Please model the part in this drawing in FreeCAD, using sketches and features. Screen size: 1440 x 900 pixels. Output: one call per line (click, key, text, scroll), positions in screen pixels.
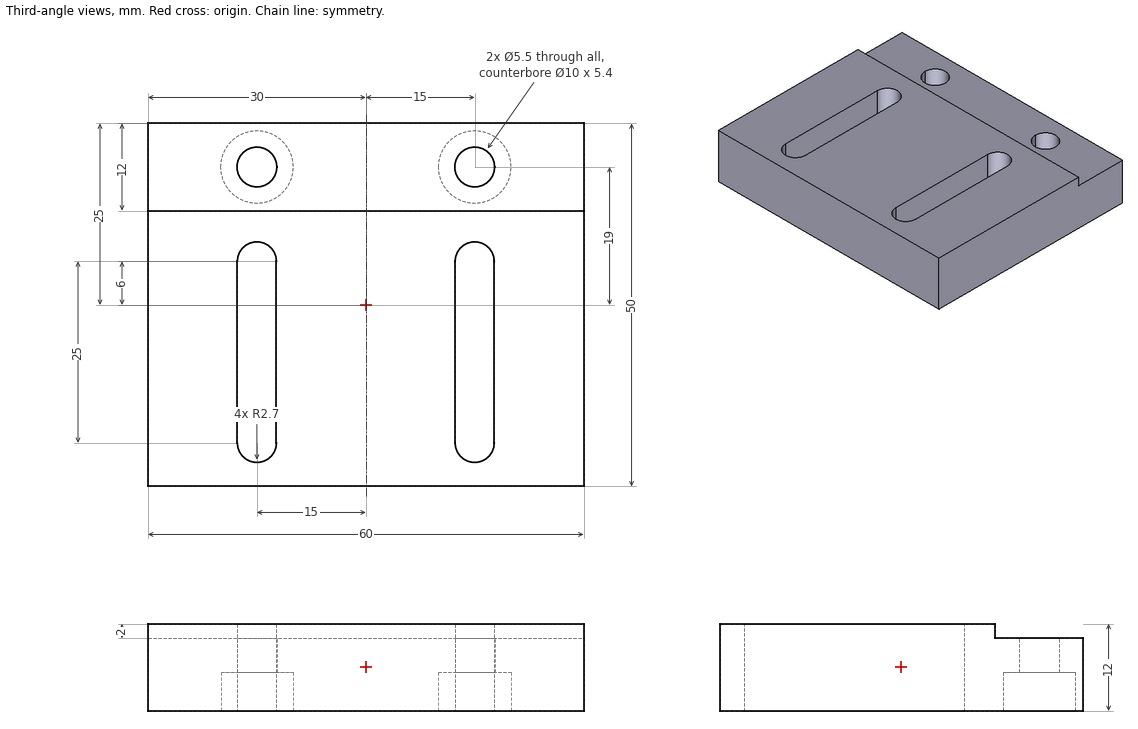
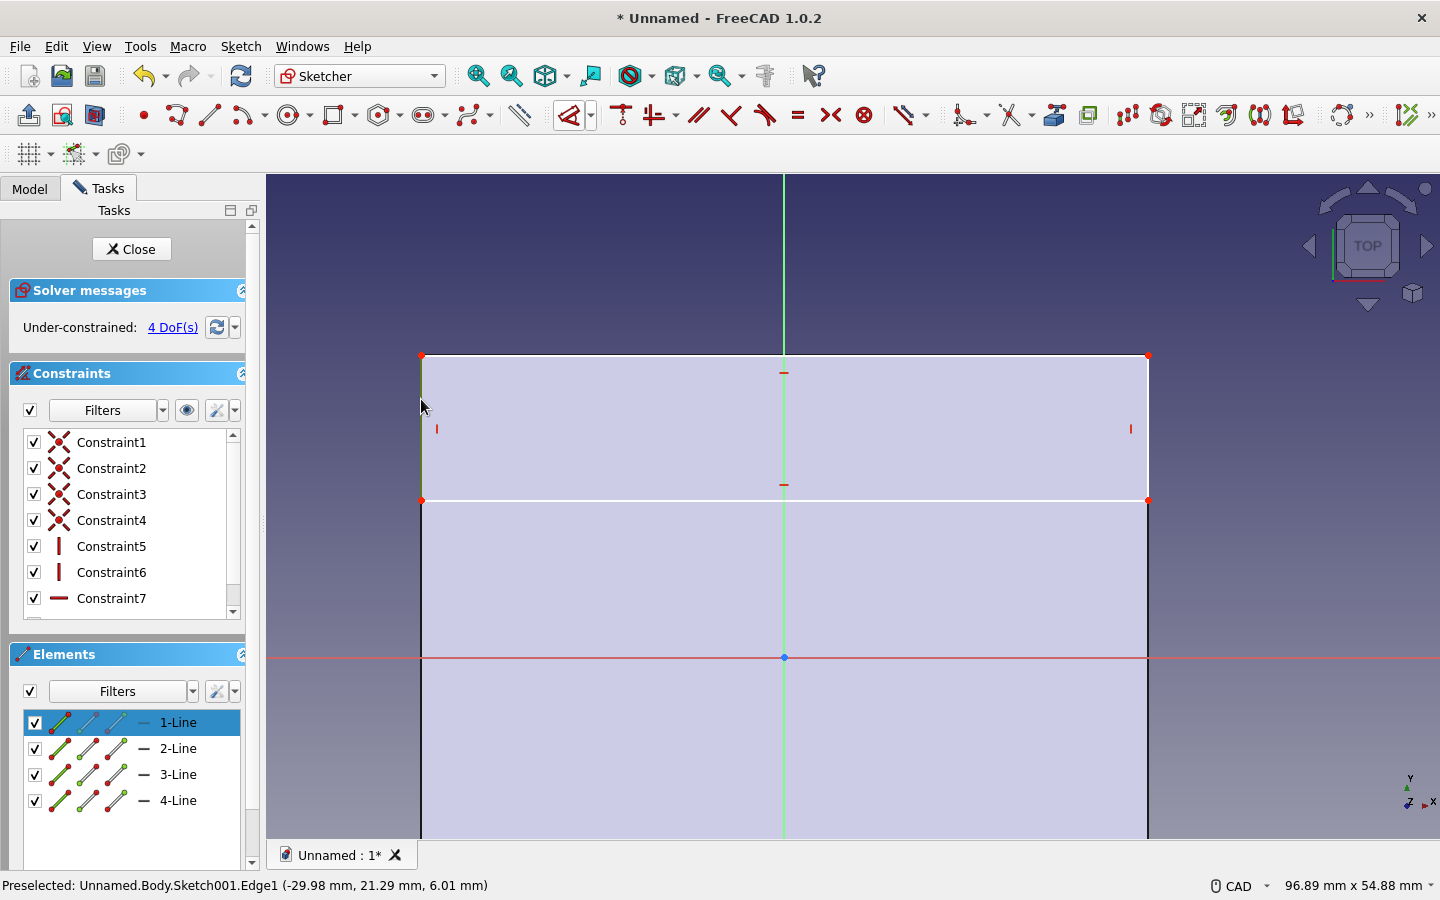
click(590, 116)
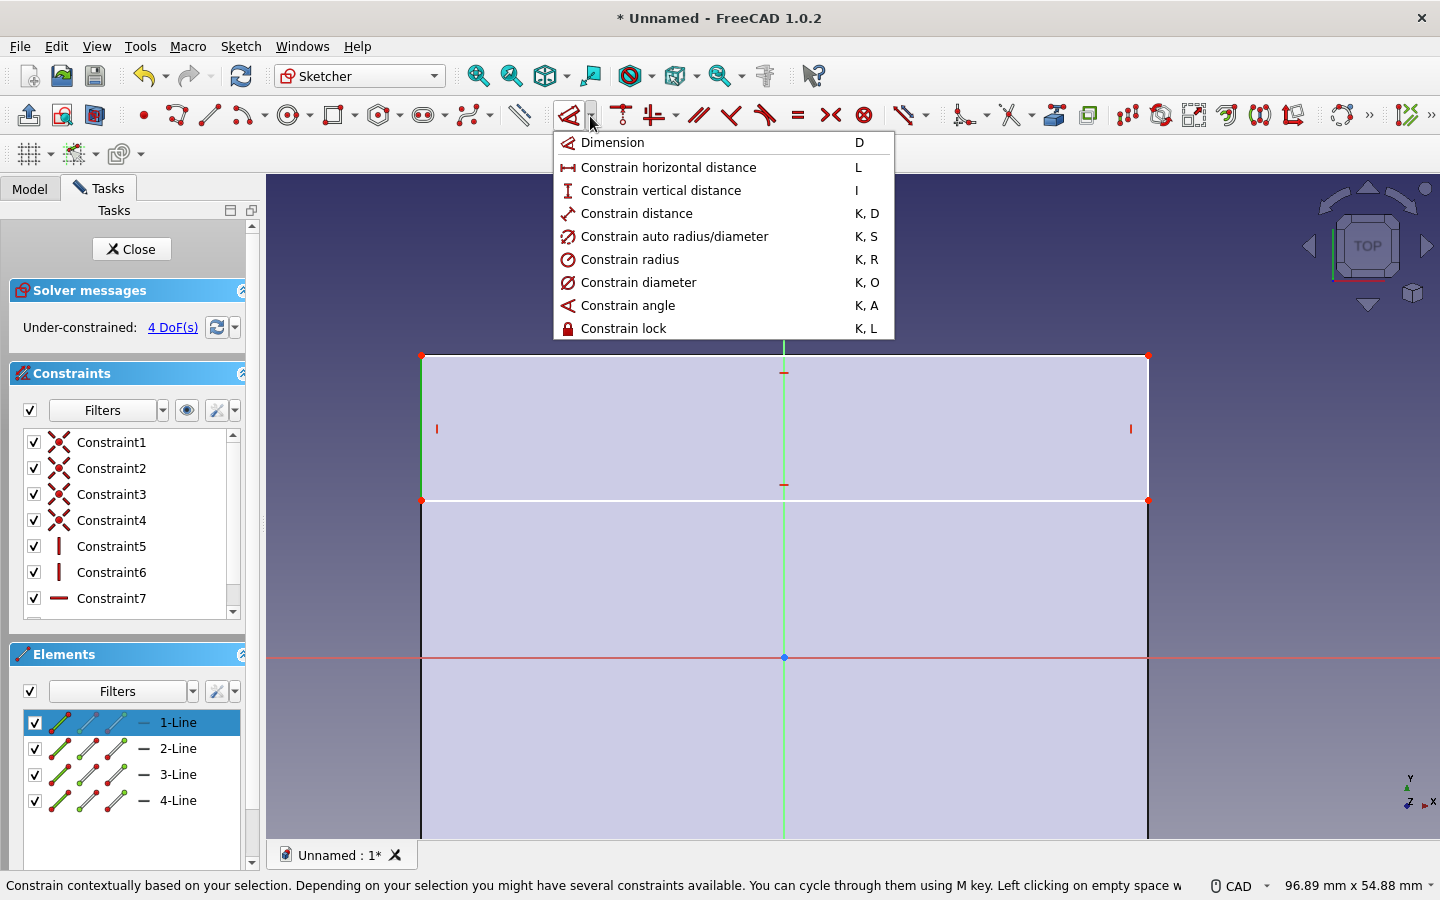
click(724, 190)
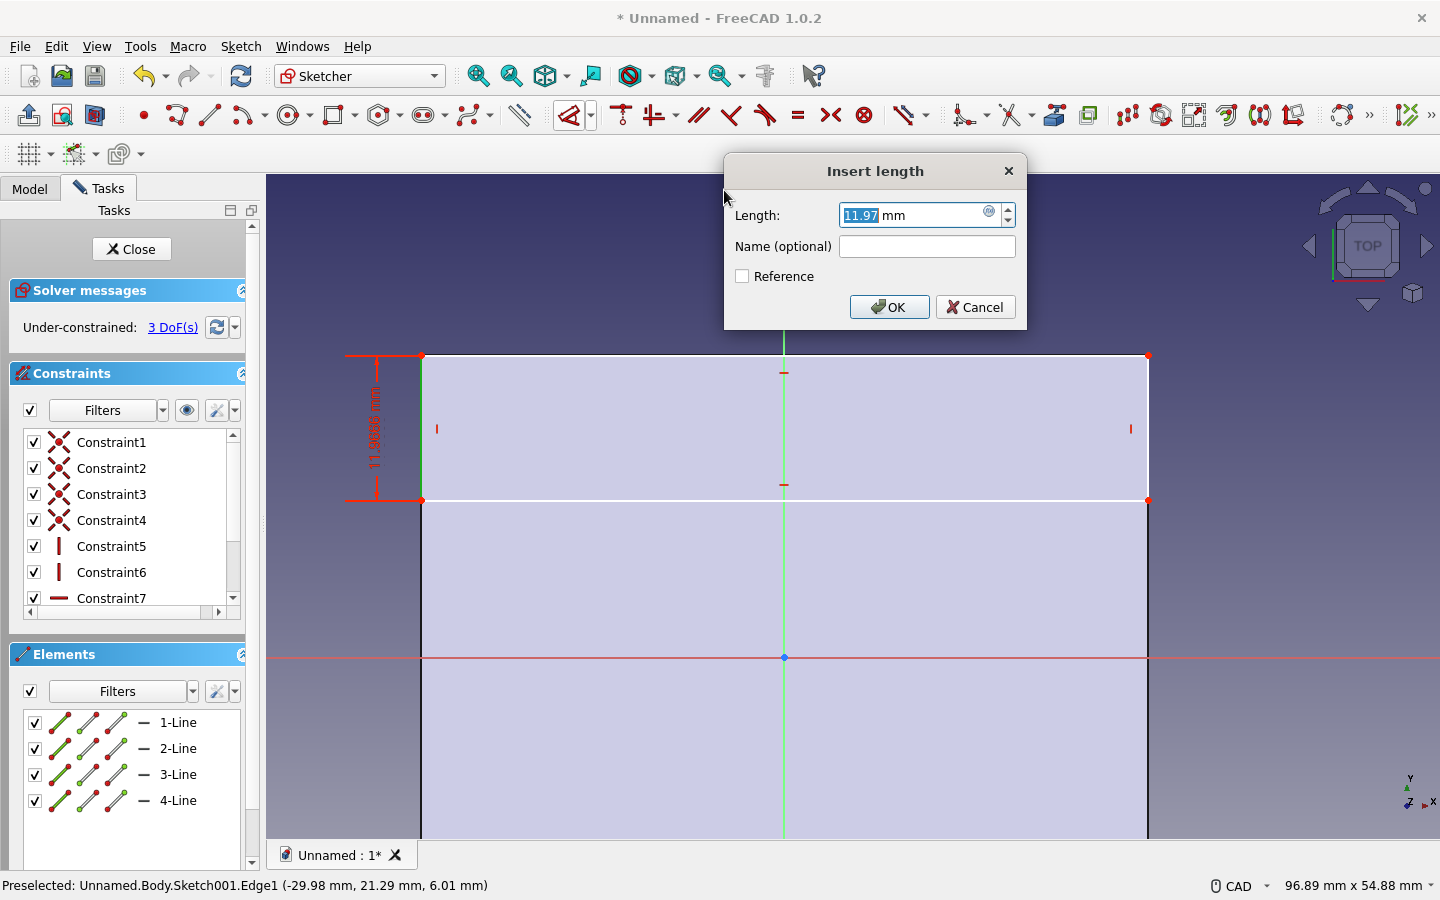
text(12)
key(Return)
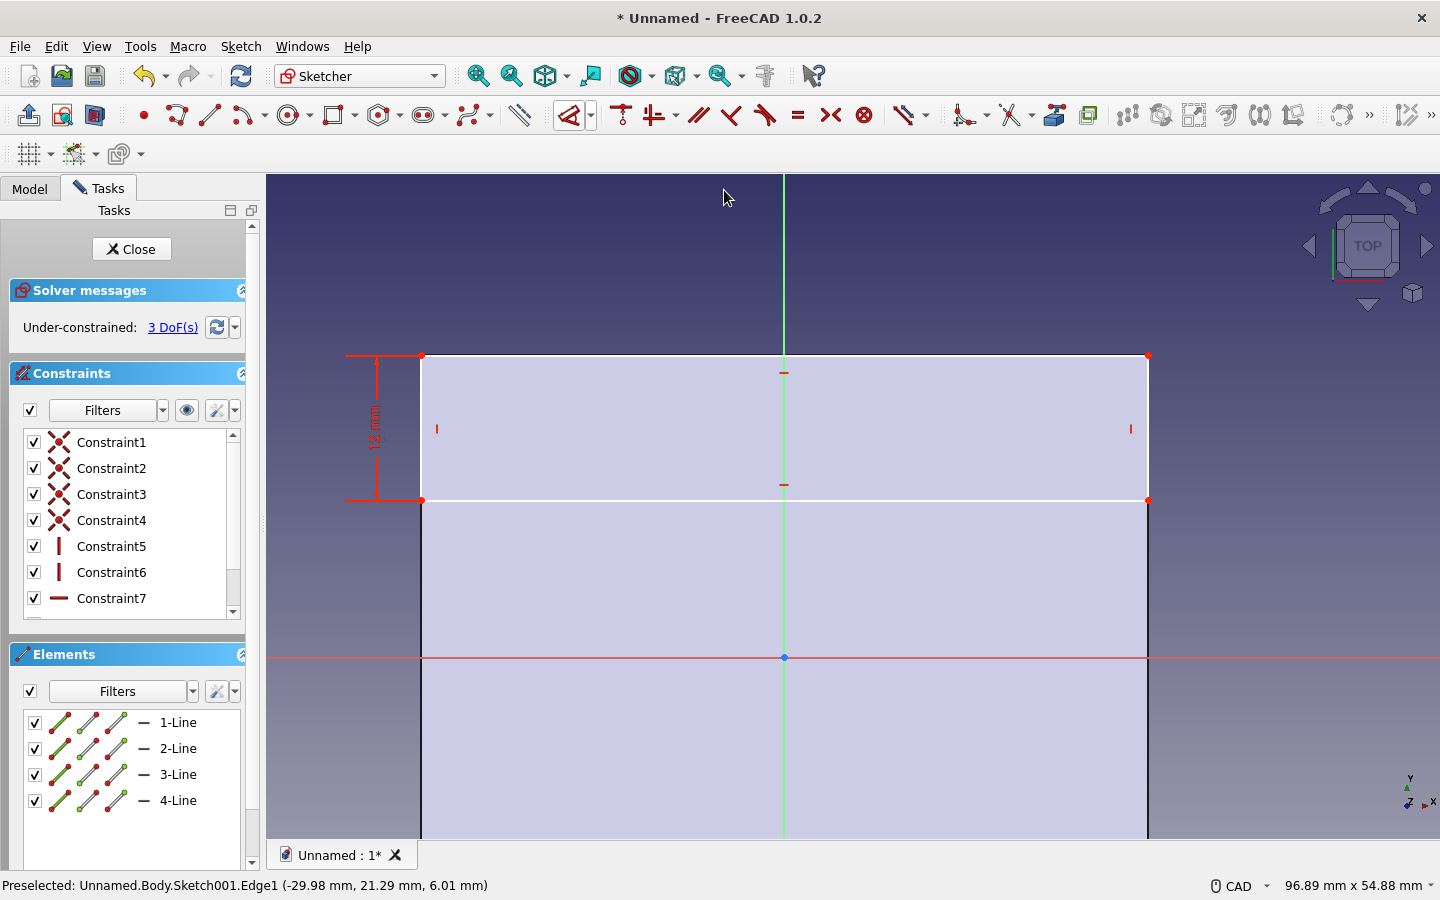
click(639, 501)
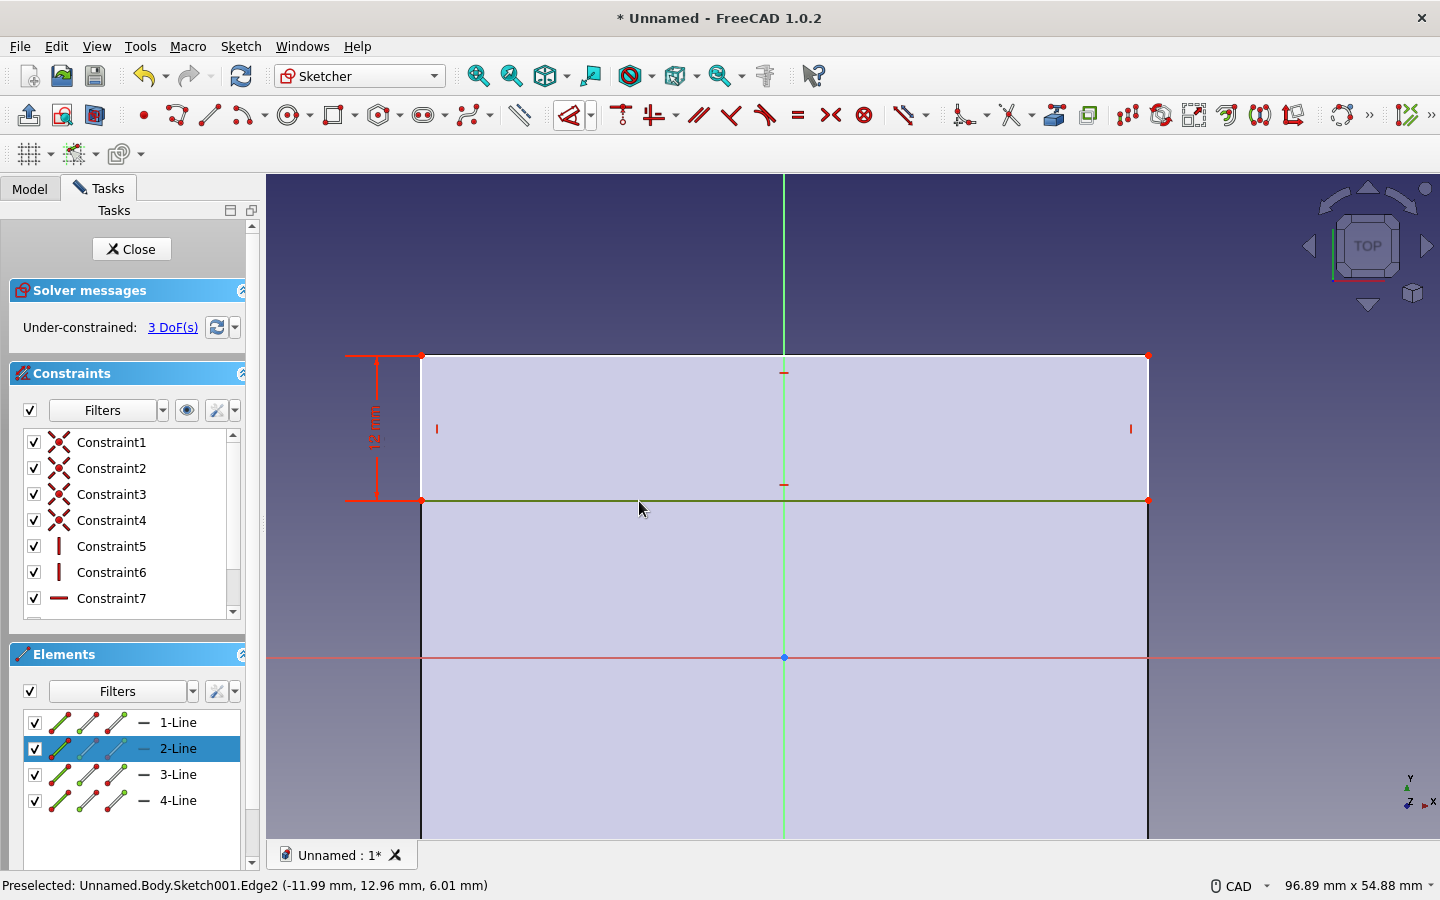
key(l)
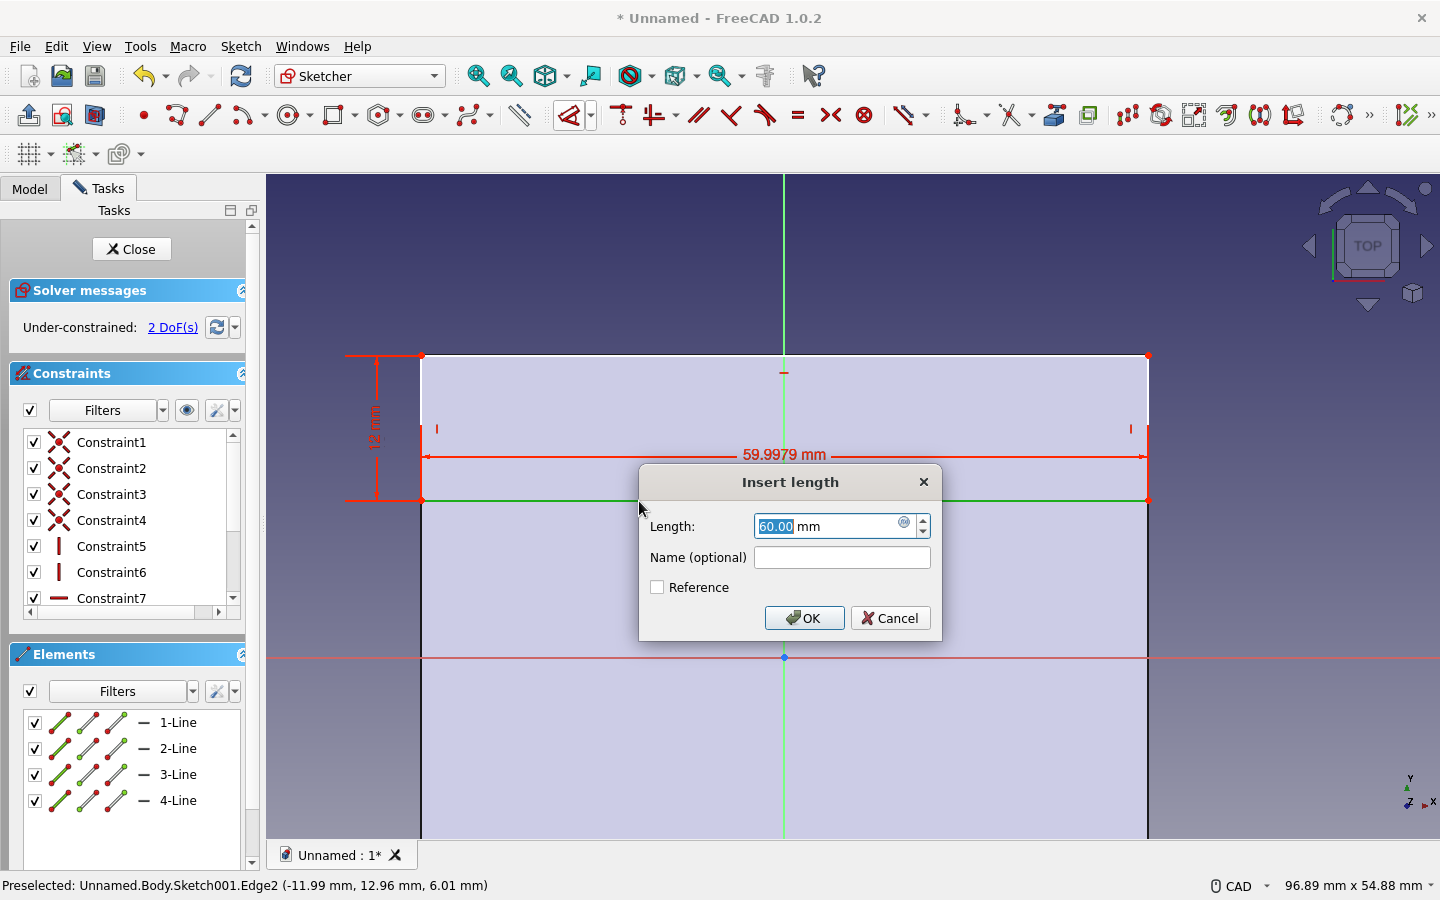
text(60)
key(Return)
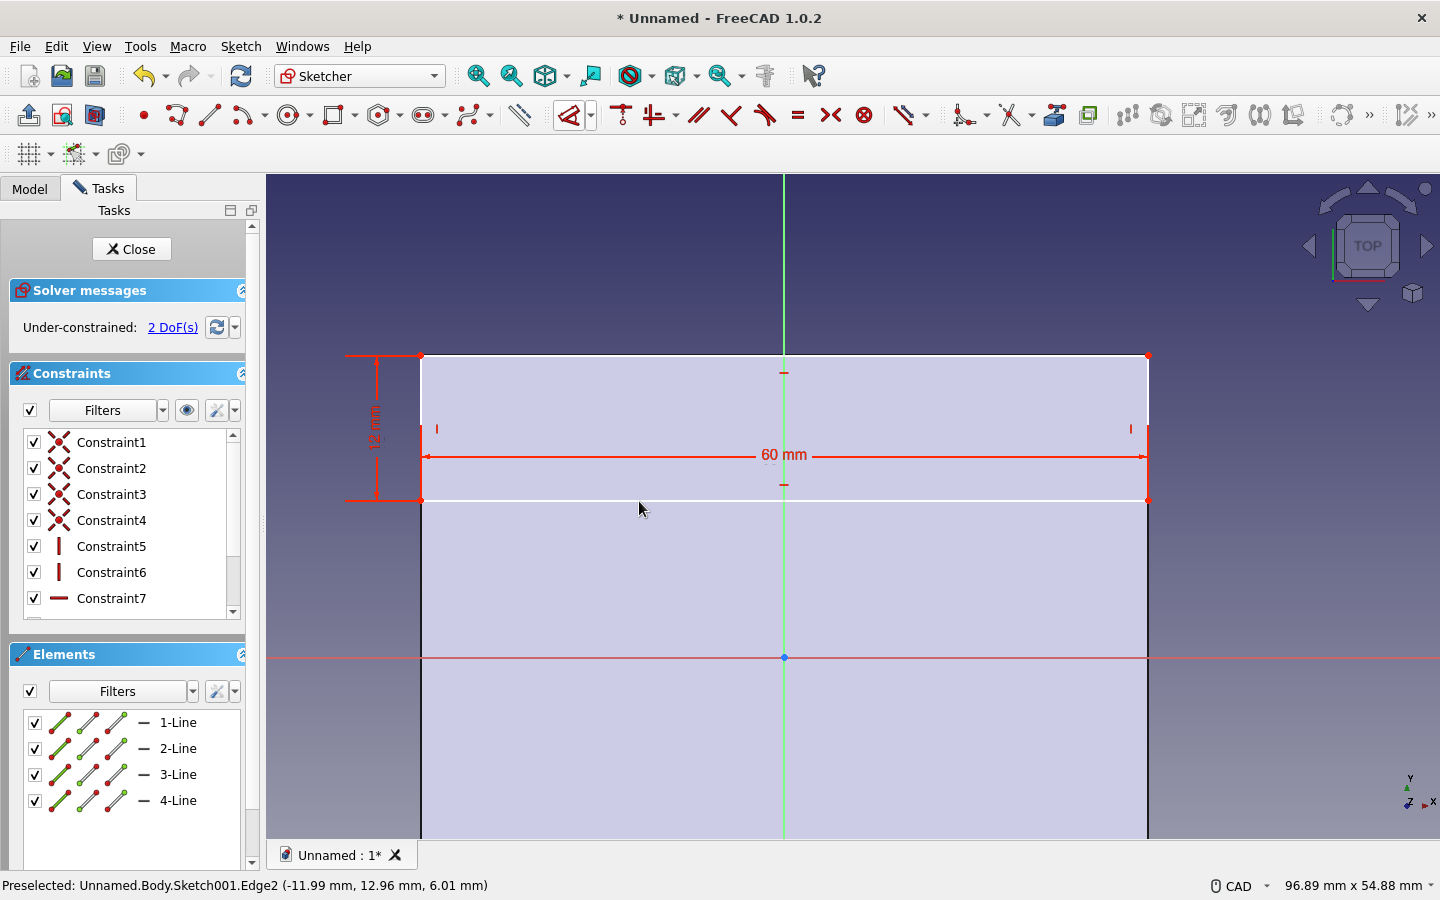
click(421, 356)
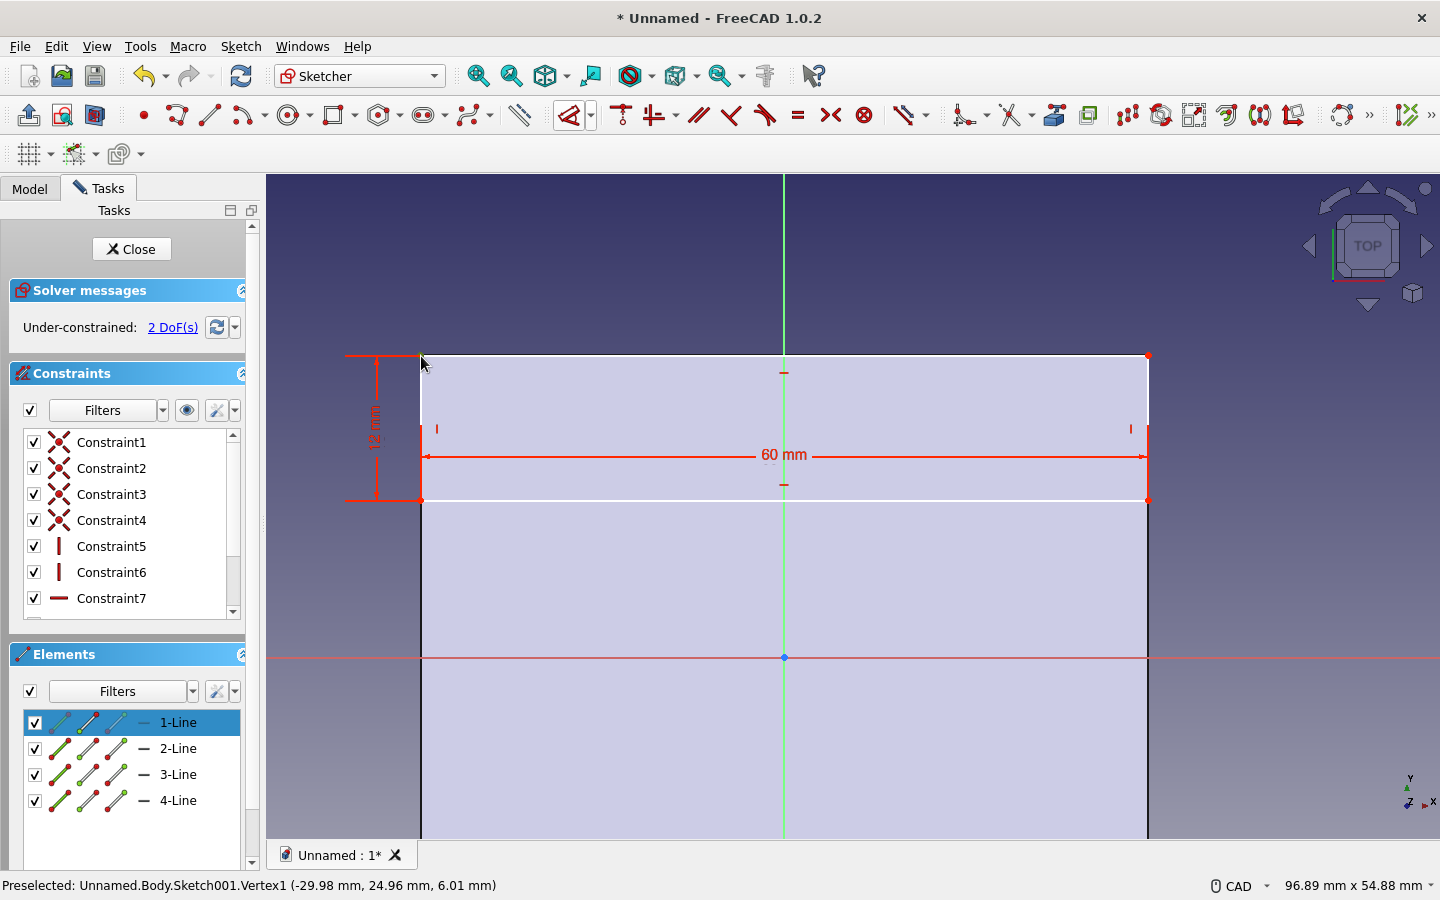
key(l)